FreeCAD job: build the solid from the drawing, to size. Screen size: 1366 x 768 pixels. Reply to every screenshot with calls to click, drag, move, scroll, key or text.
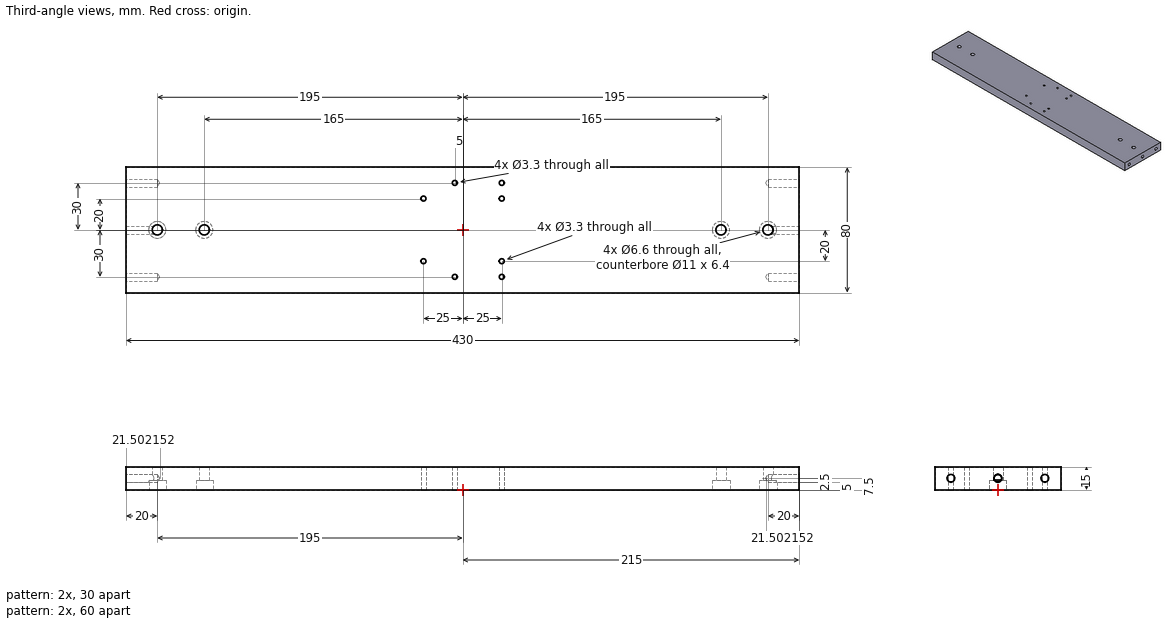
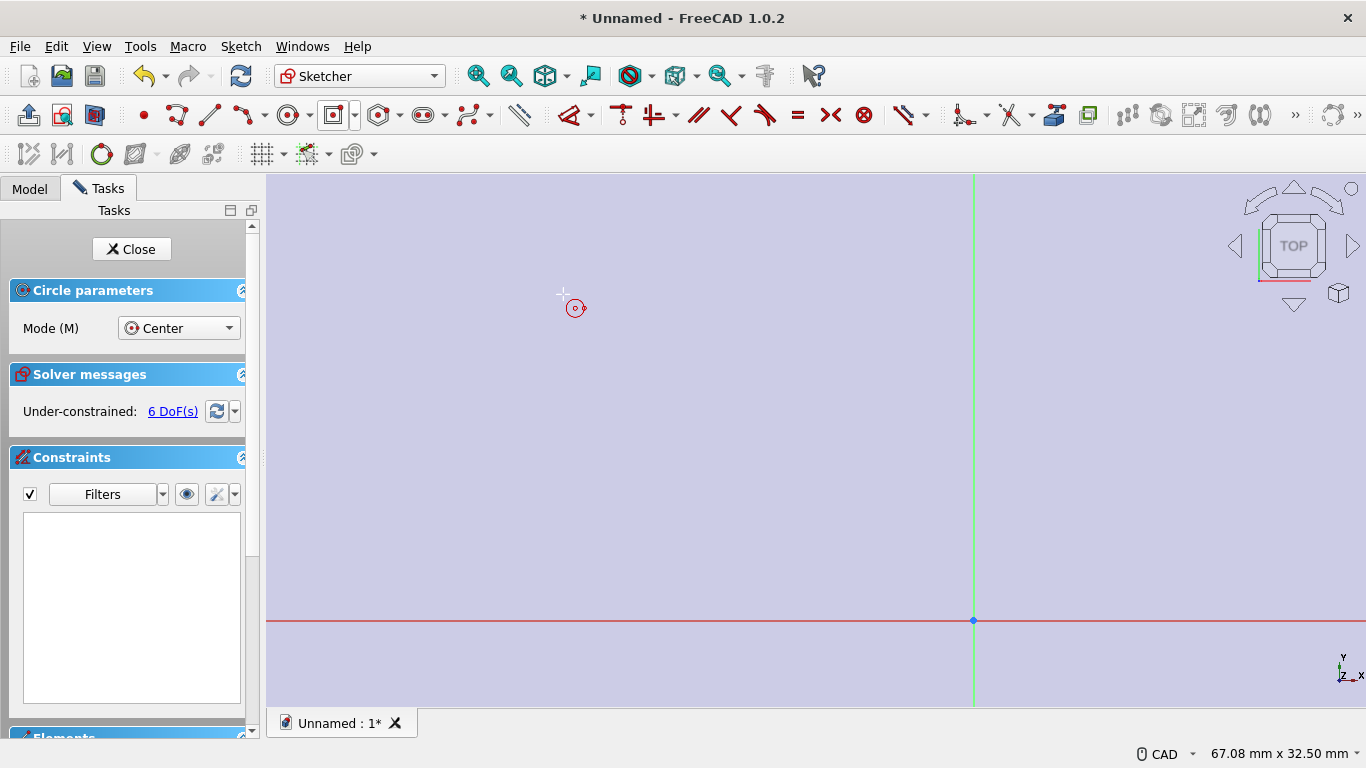
click(564, 293)
click(583, 274)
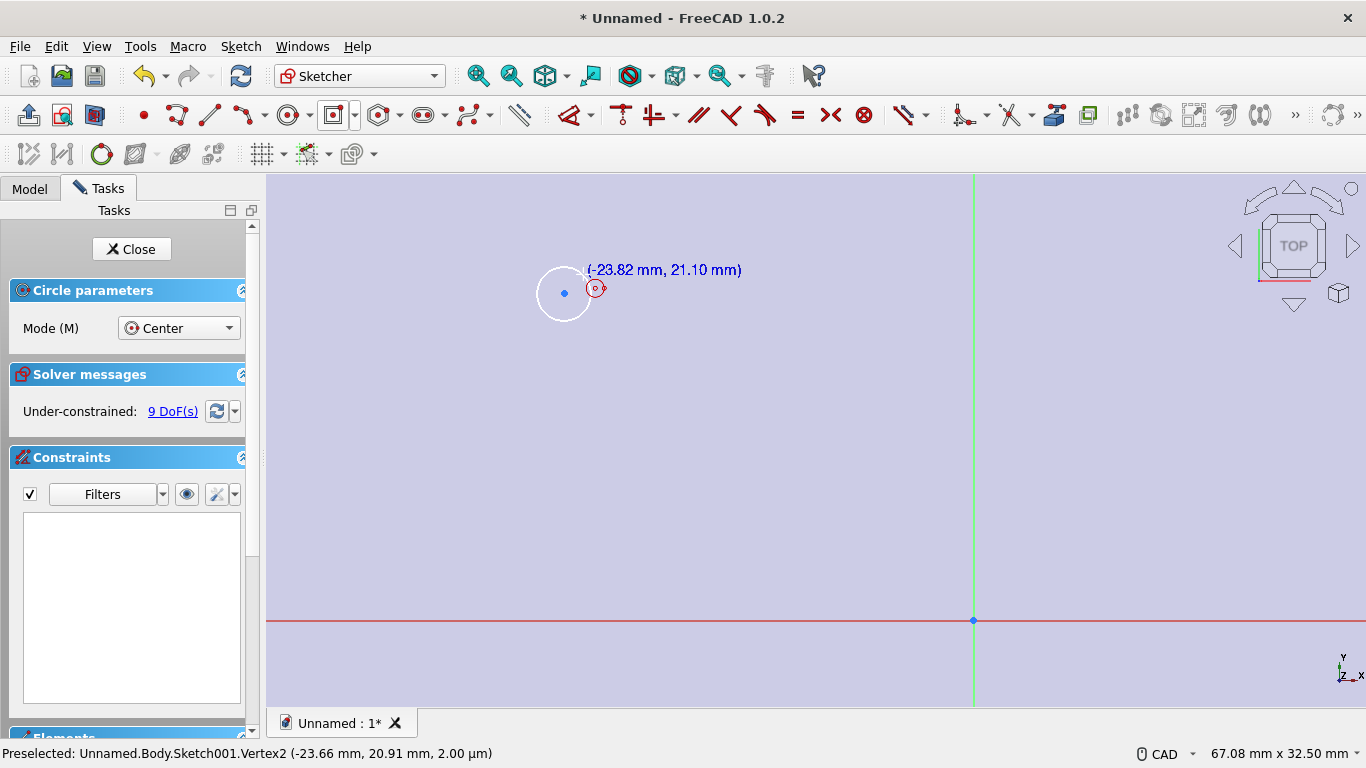
scroll(563, 293, down, 4)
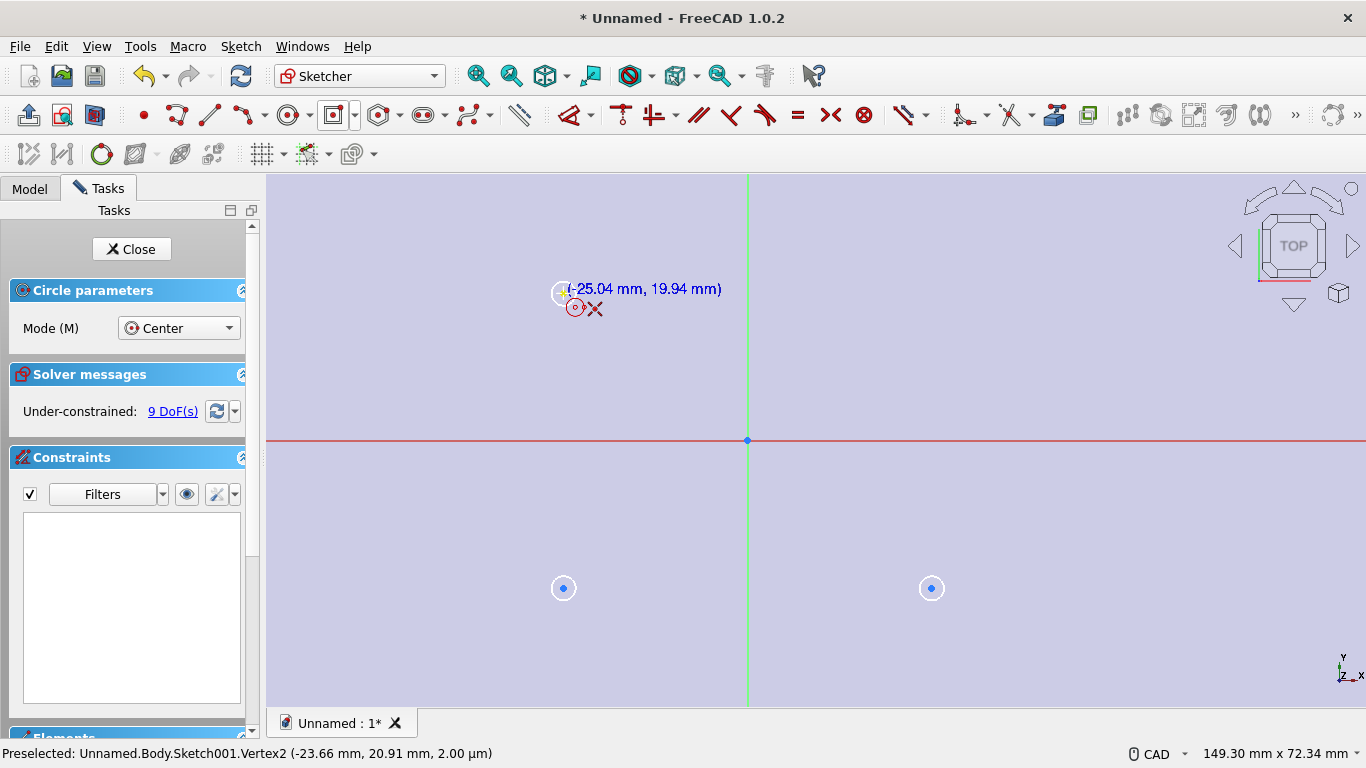
scroll(932, 293, up, 4)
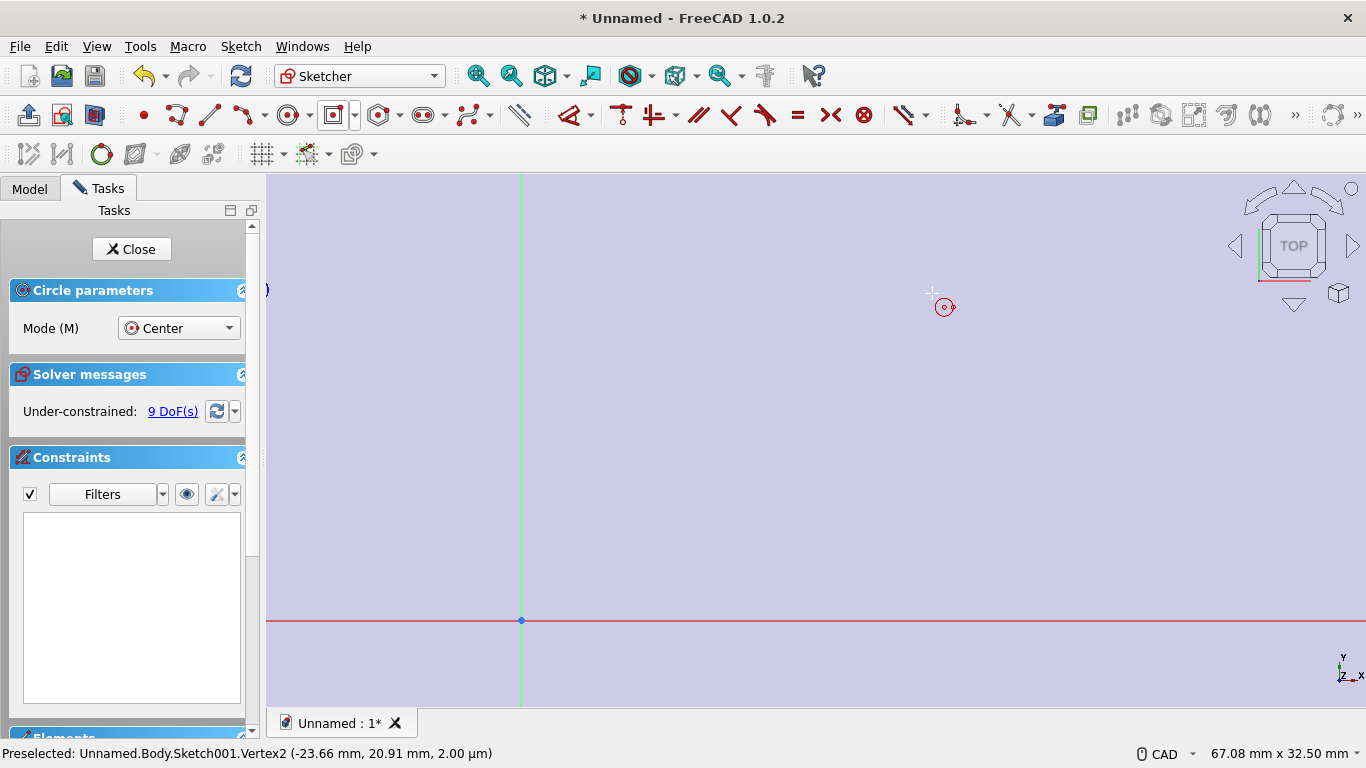
click(931, 293)
click(950, 274)
key(Escape)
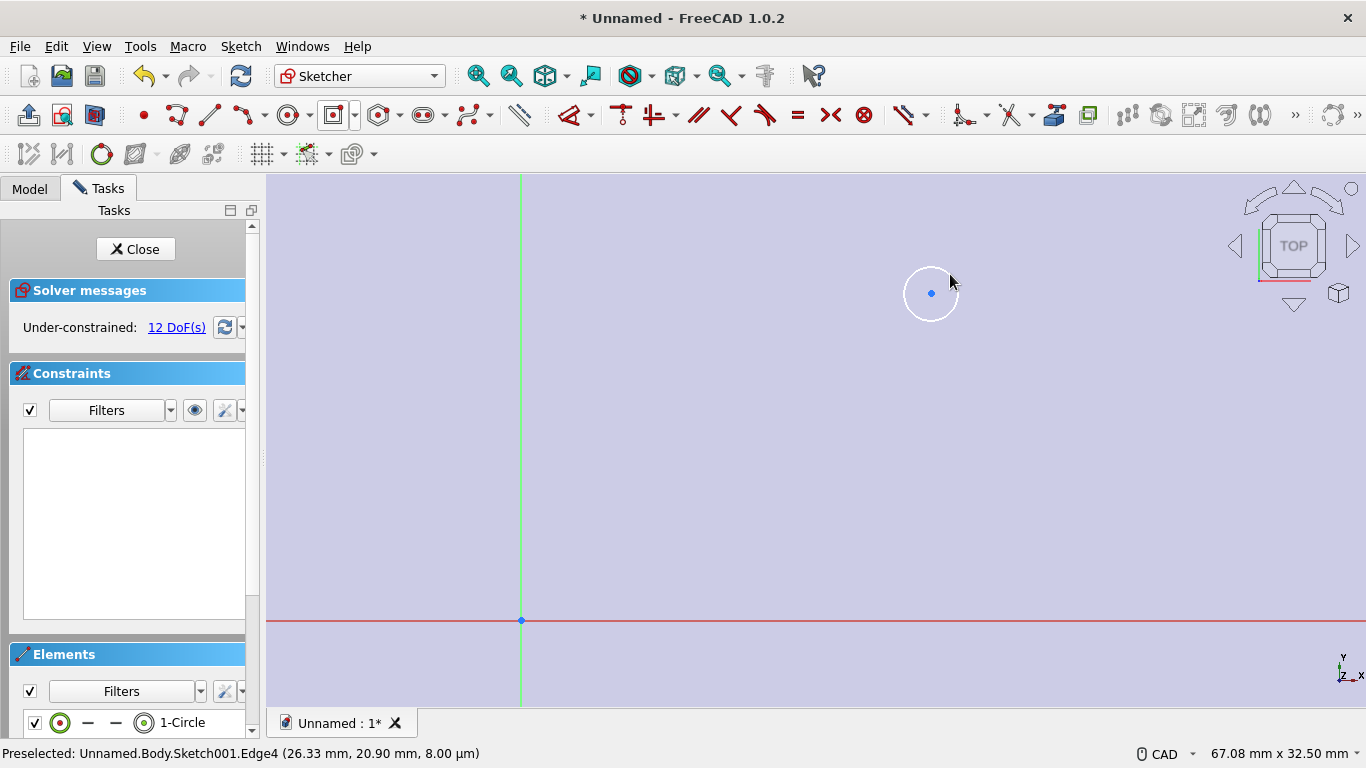
scroll(932, 293, down, 4)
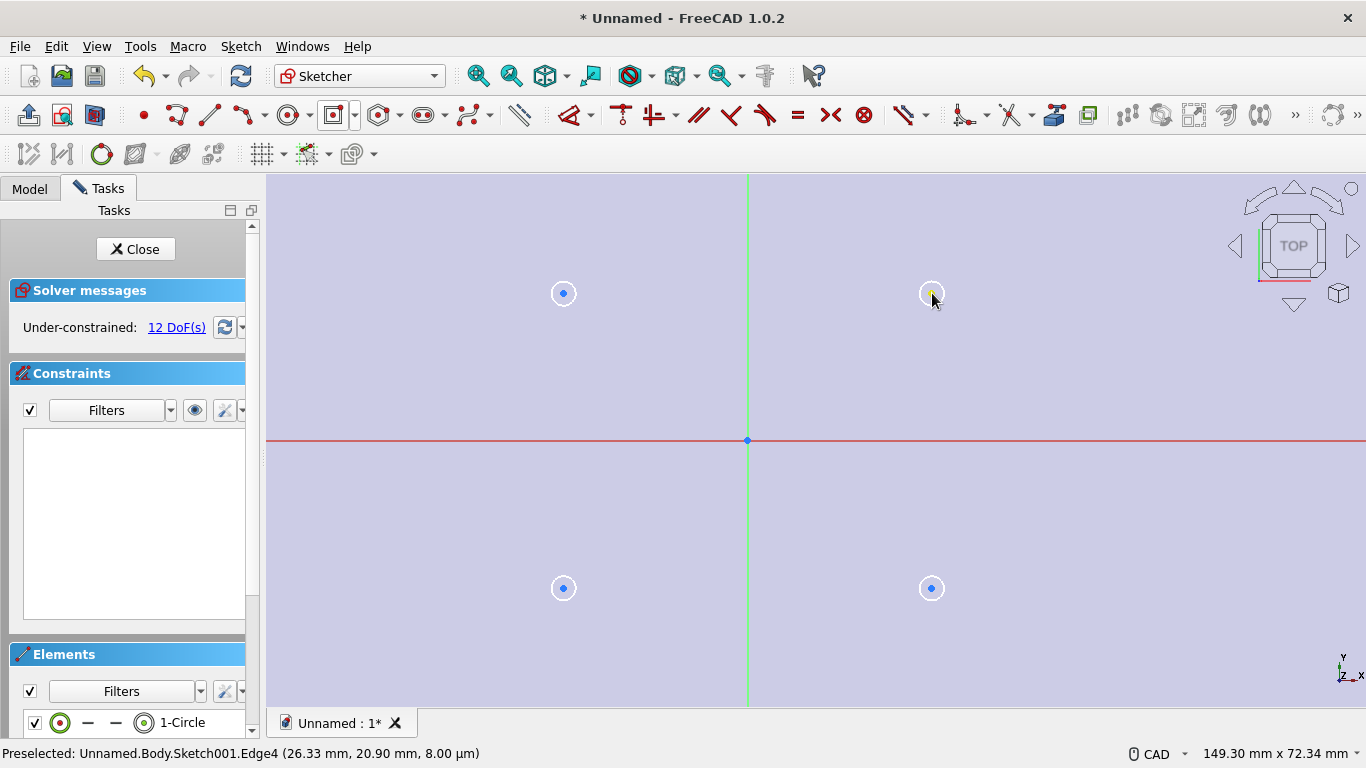
click(940, 580)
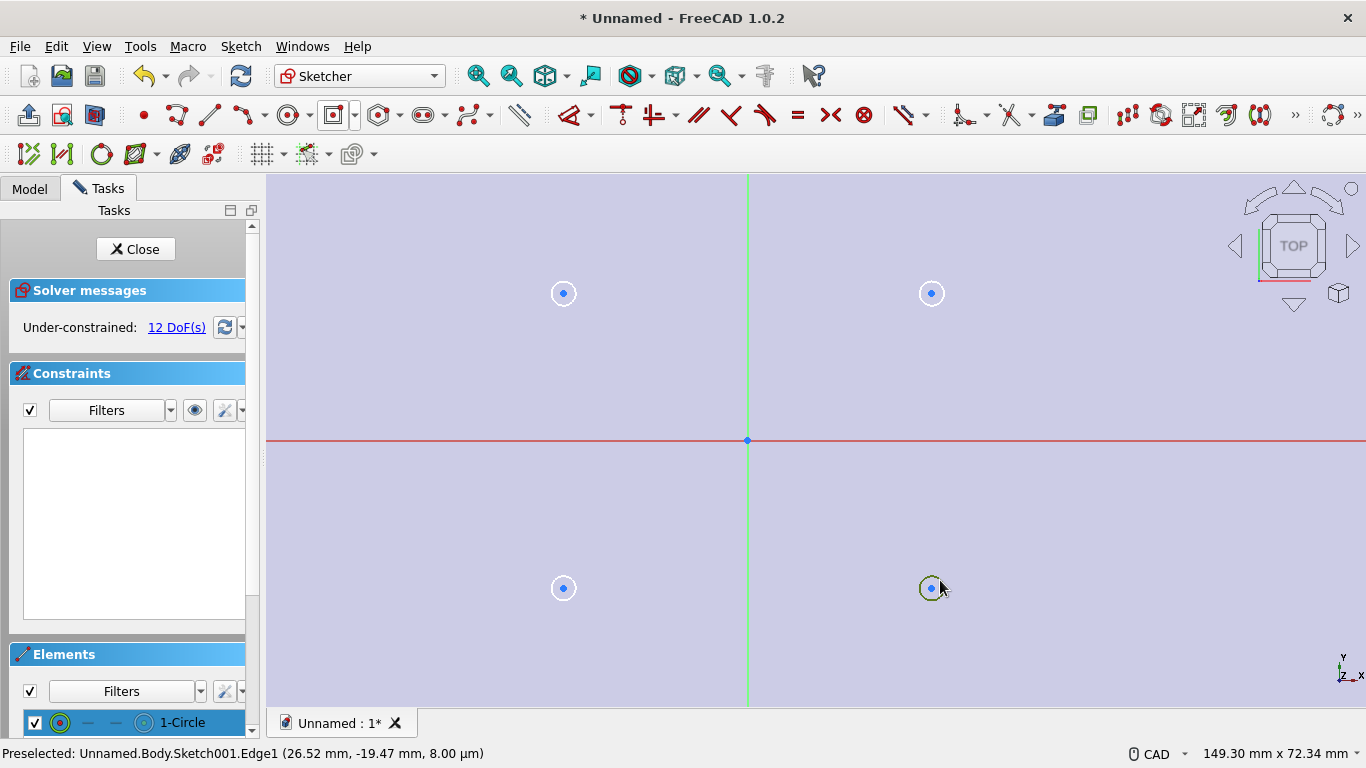
click(572, 580)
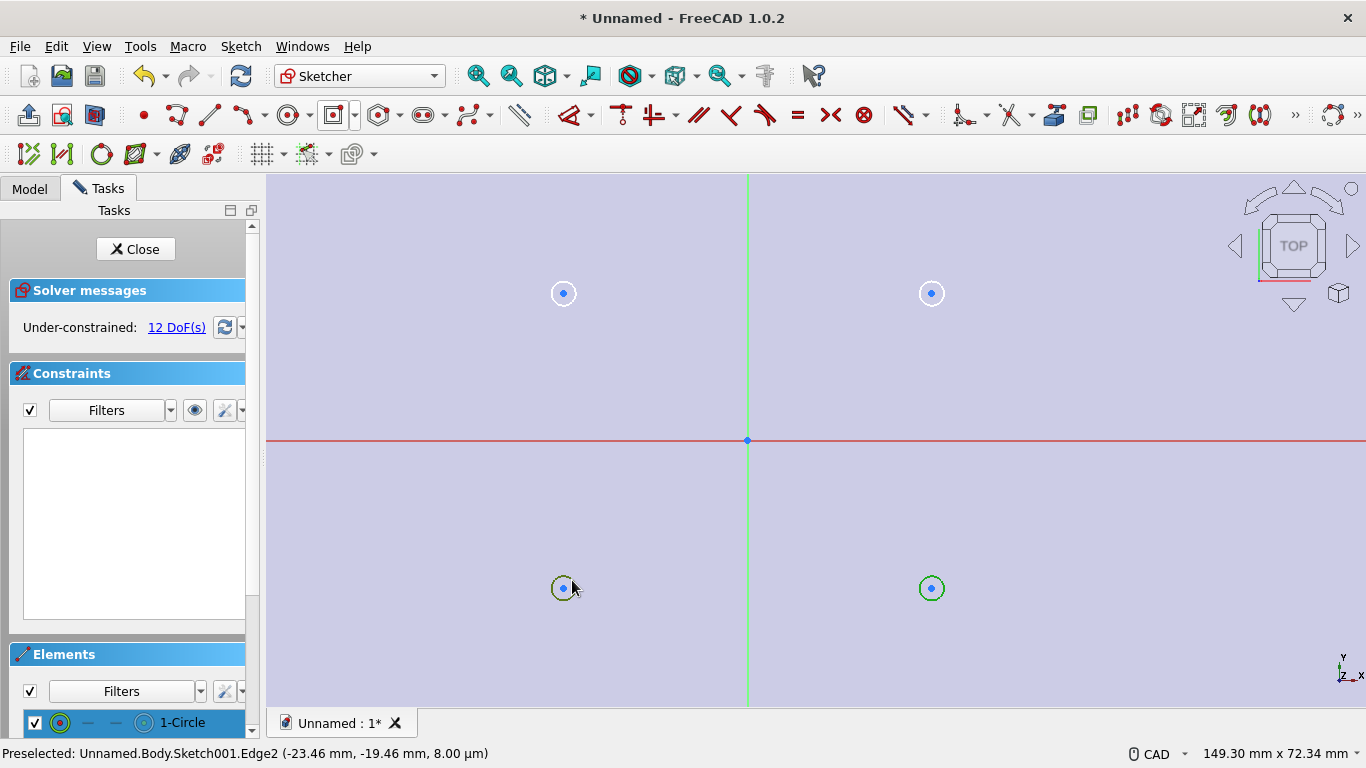
click(572, 285)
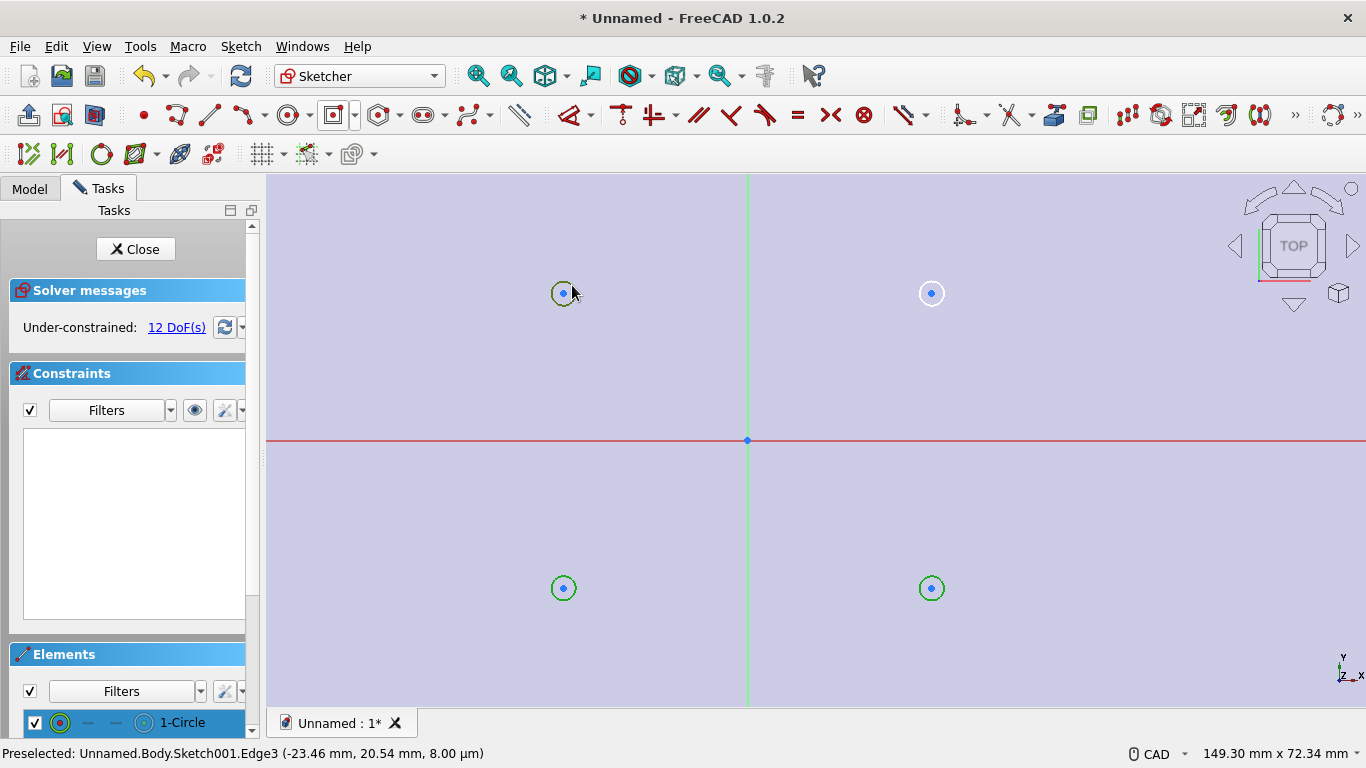
click(940, 285)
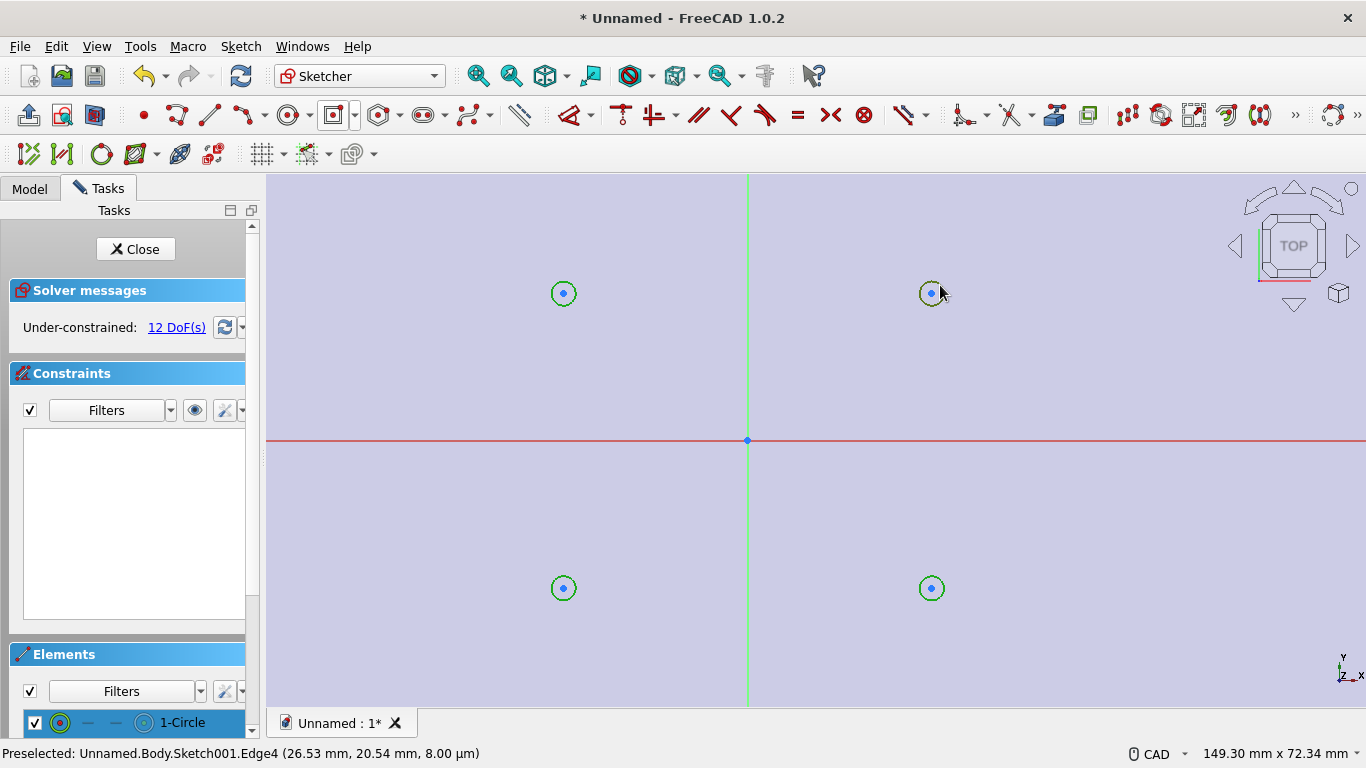
click(798, 116)